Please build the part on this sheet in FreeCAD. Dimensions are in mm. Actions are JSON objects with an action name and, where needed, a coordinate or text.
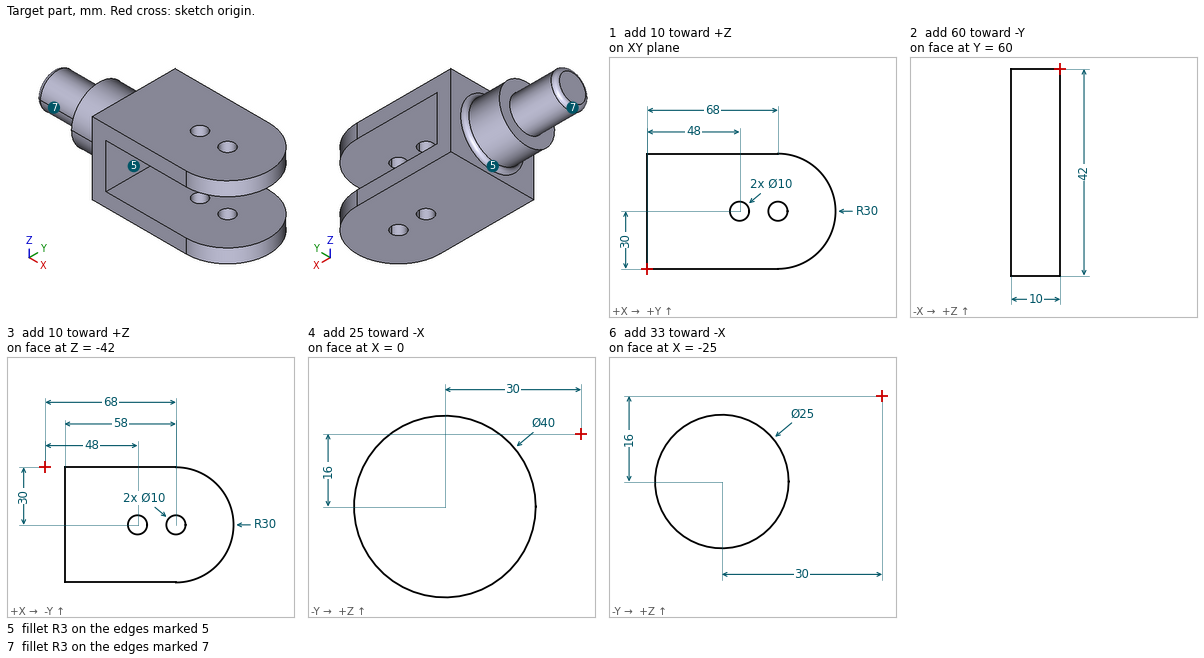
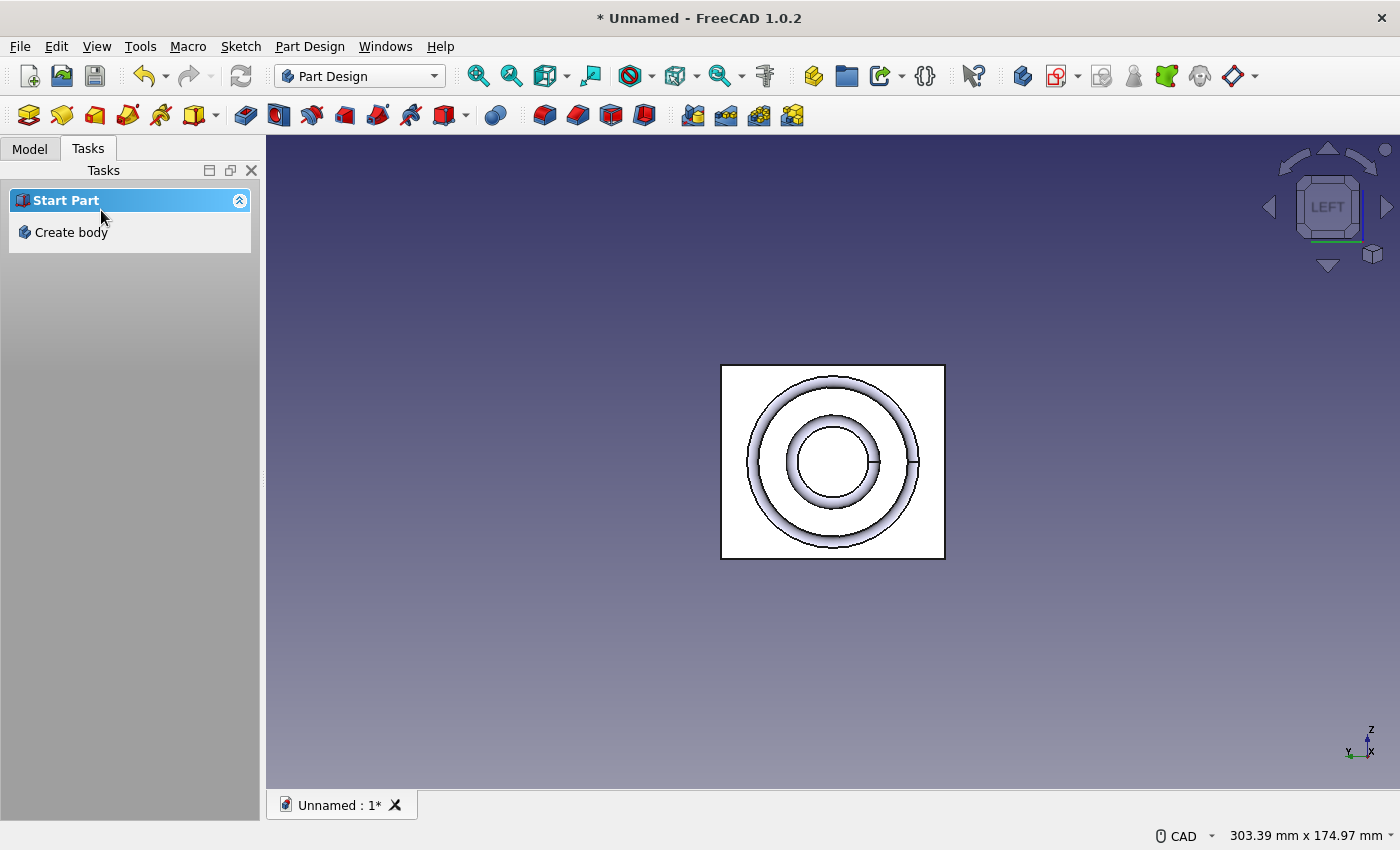
{"action": "key", "text": "0"}